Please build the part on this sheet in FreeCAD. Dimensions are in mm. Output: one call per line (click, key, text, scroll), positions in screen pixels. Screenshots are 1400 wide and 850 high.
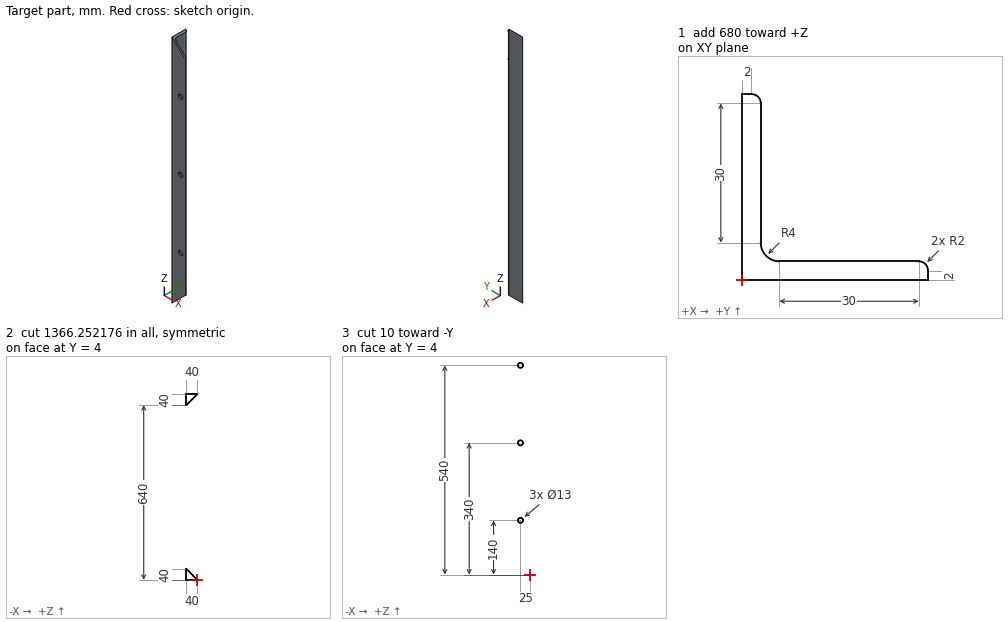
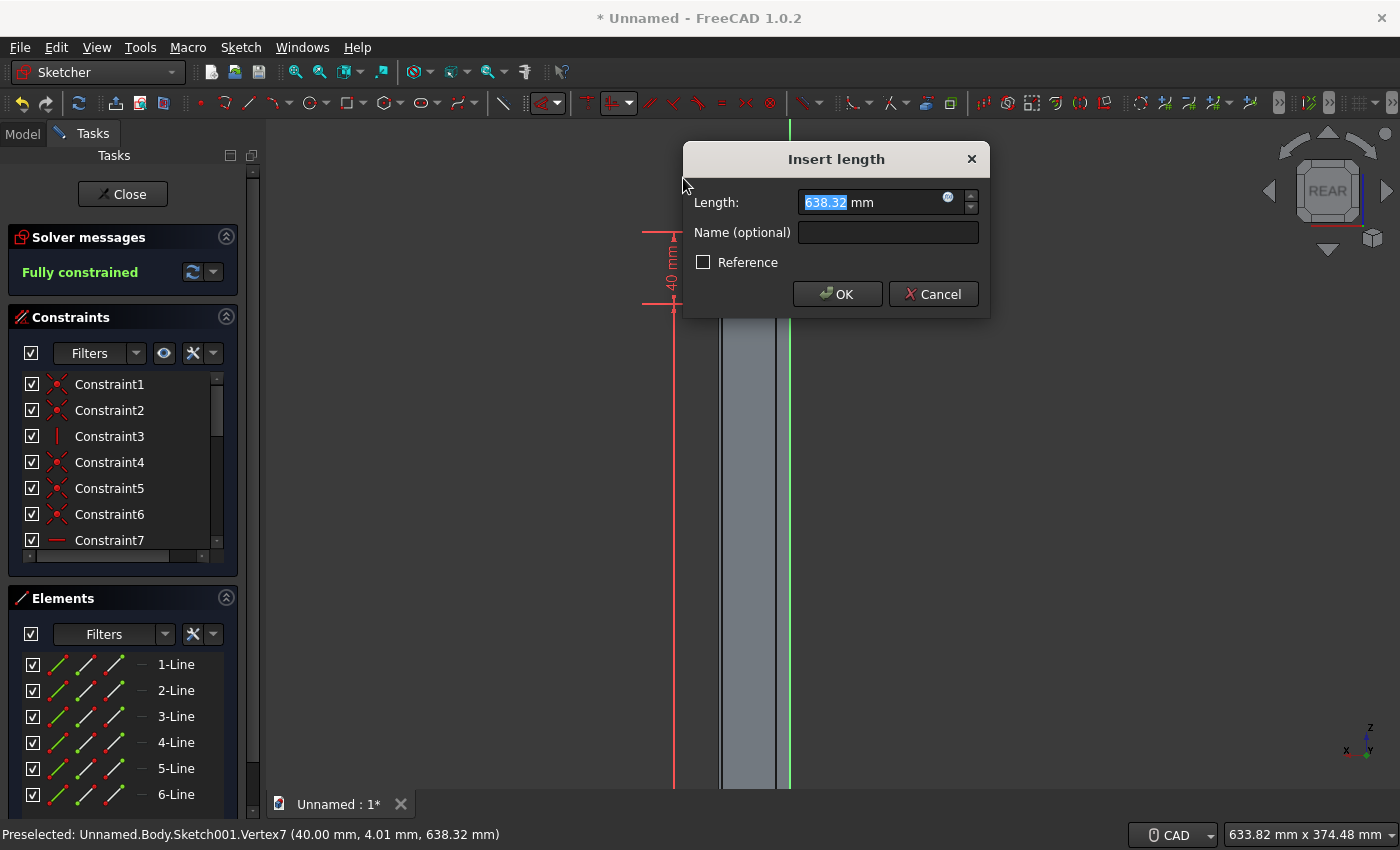
text(640)
key(Return)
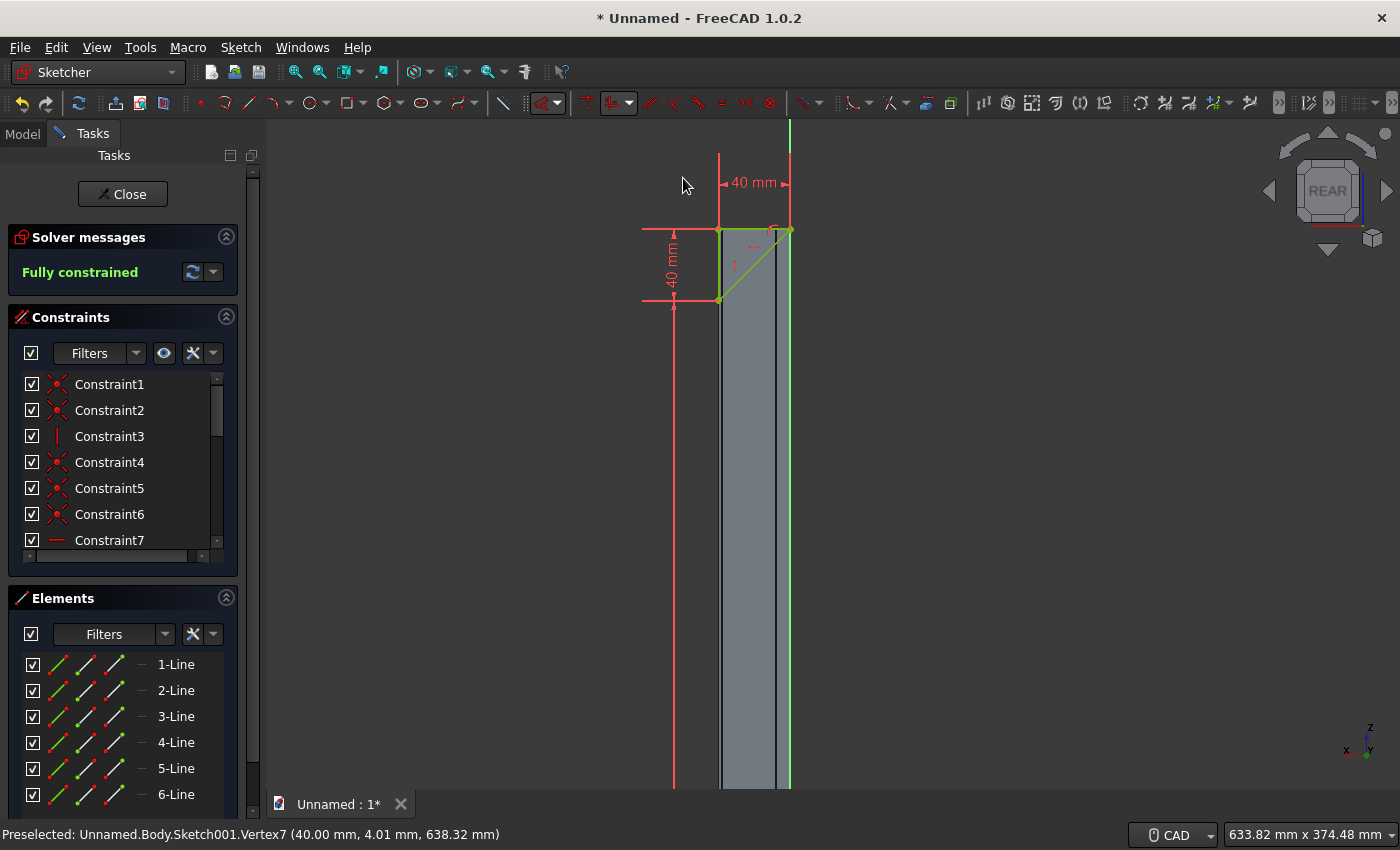
click(123, 194)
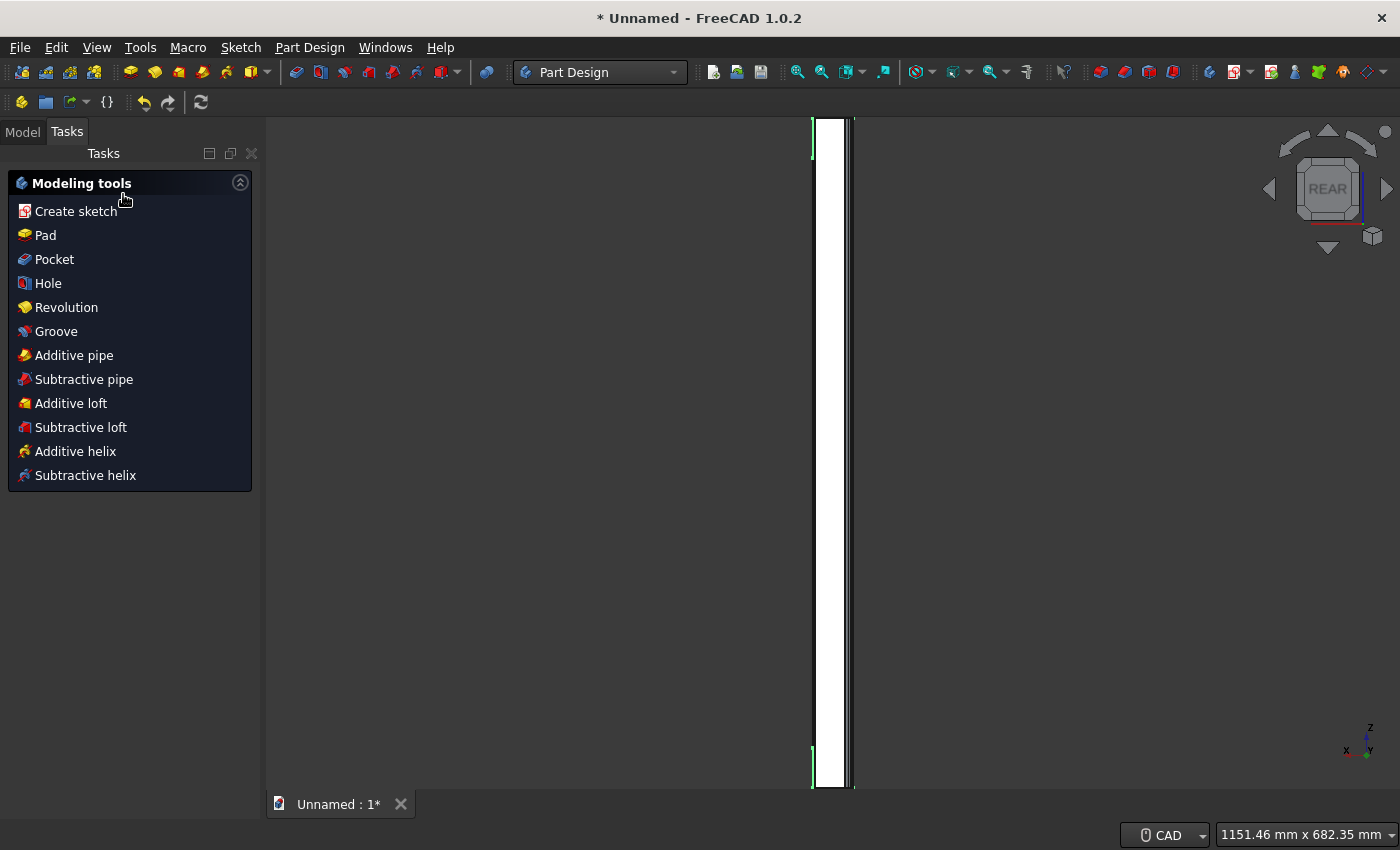
click(298, 72)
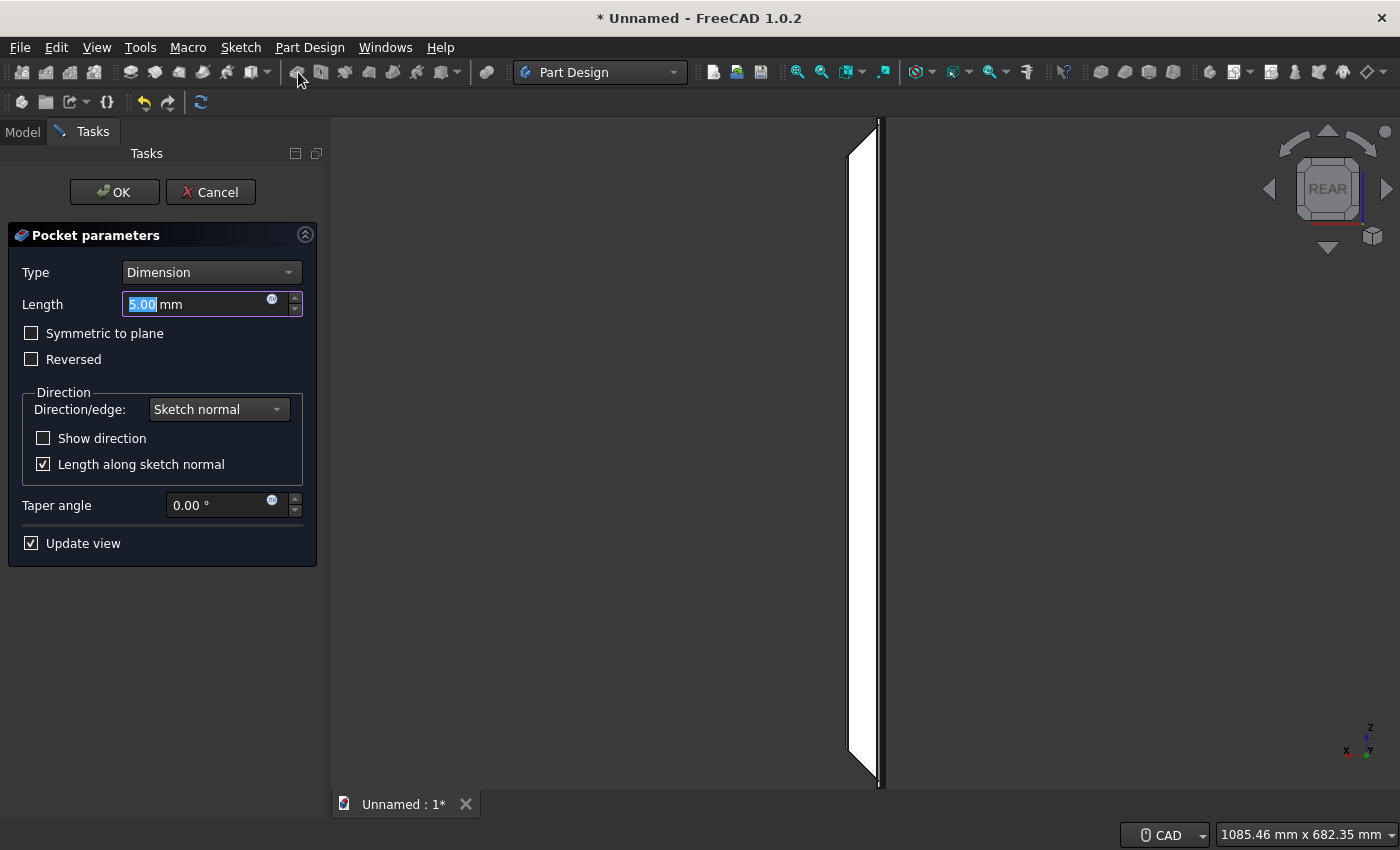
text(1366.252176)
key(Tab)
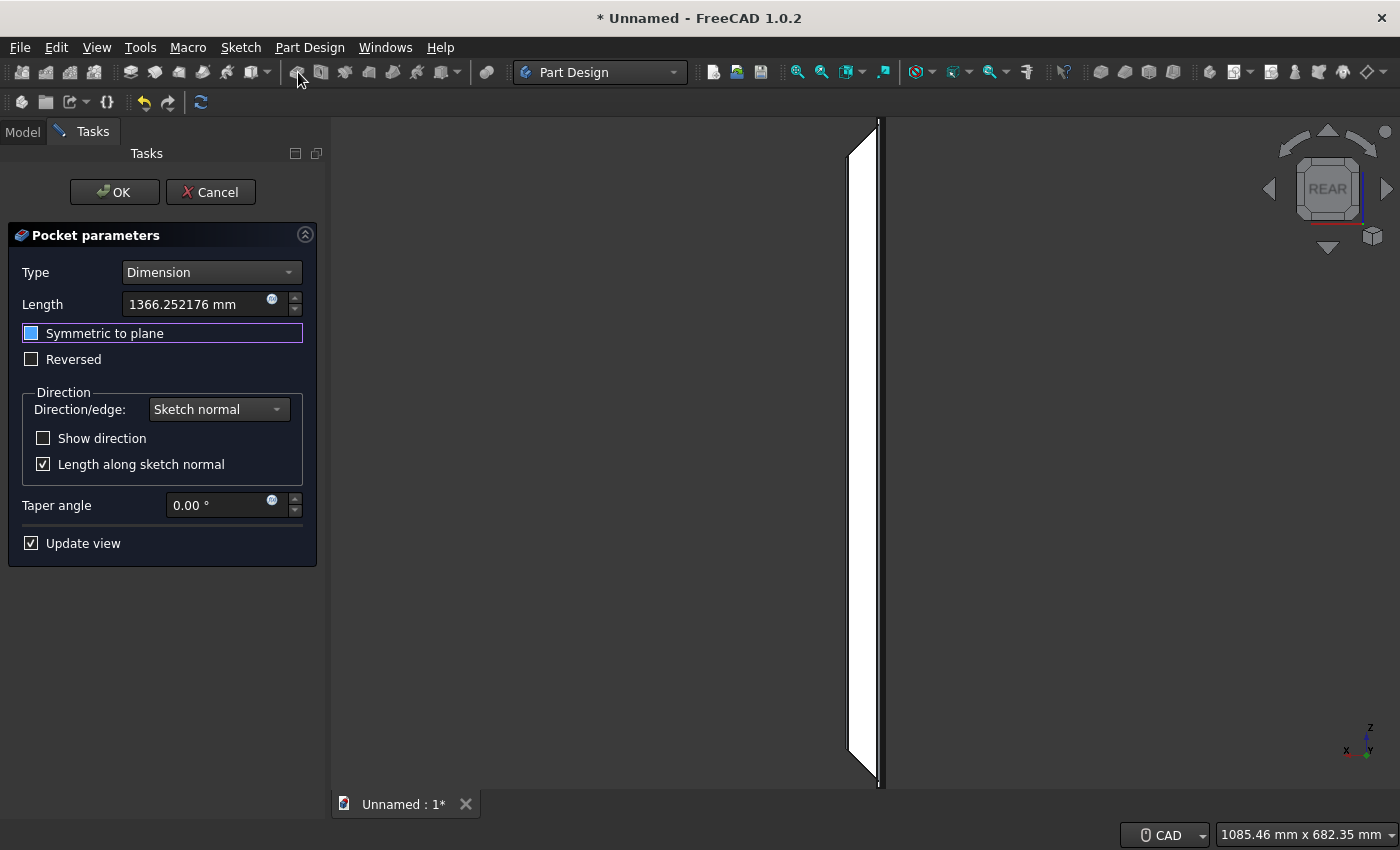
click(30, 333)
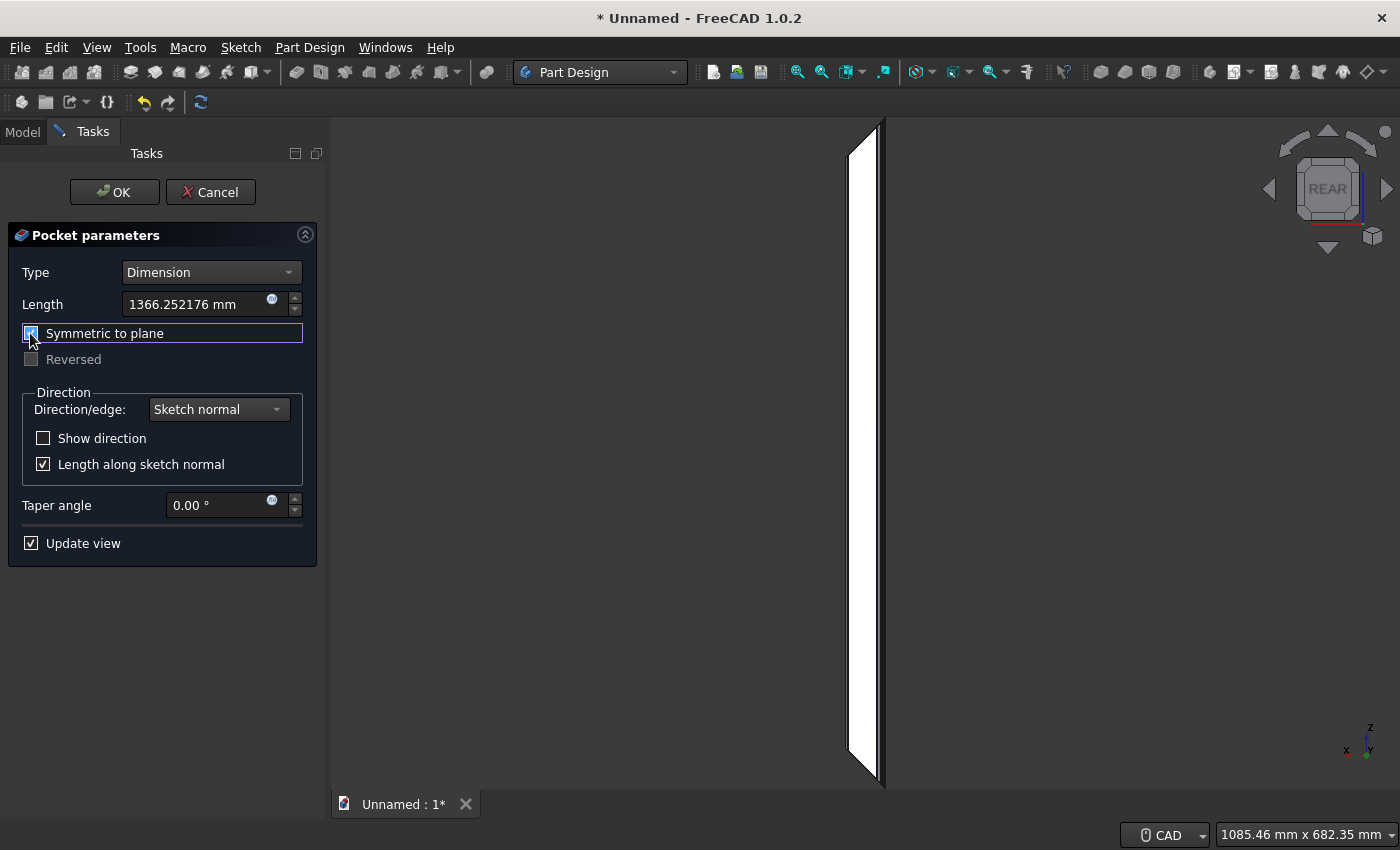
click(115, 192)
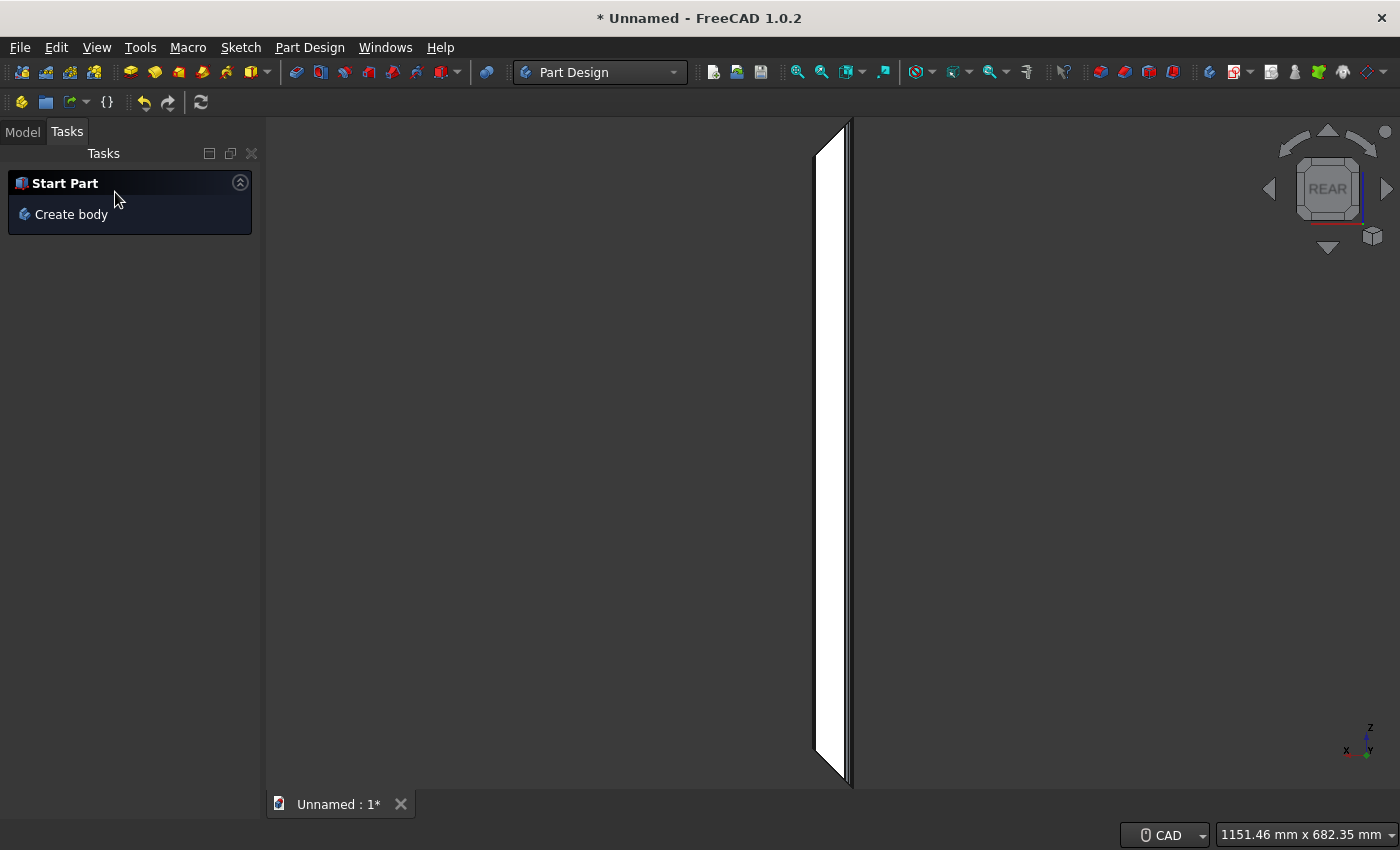
click(830, 172)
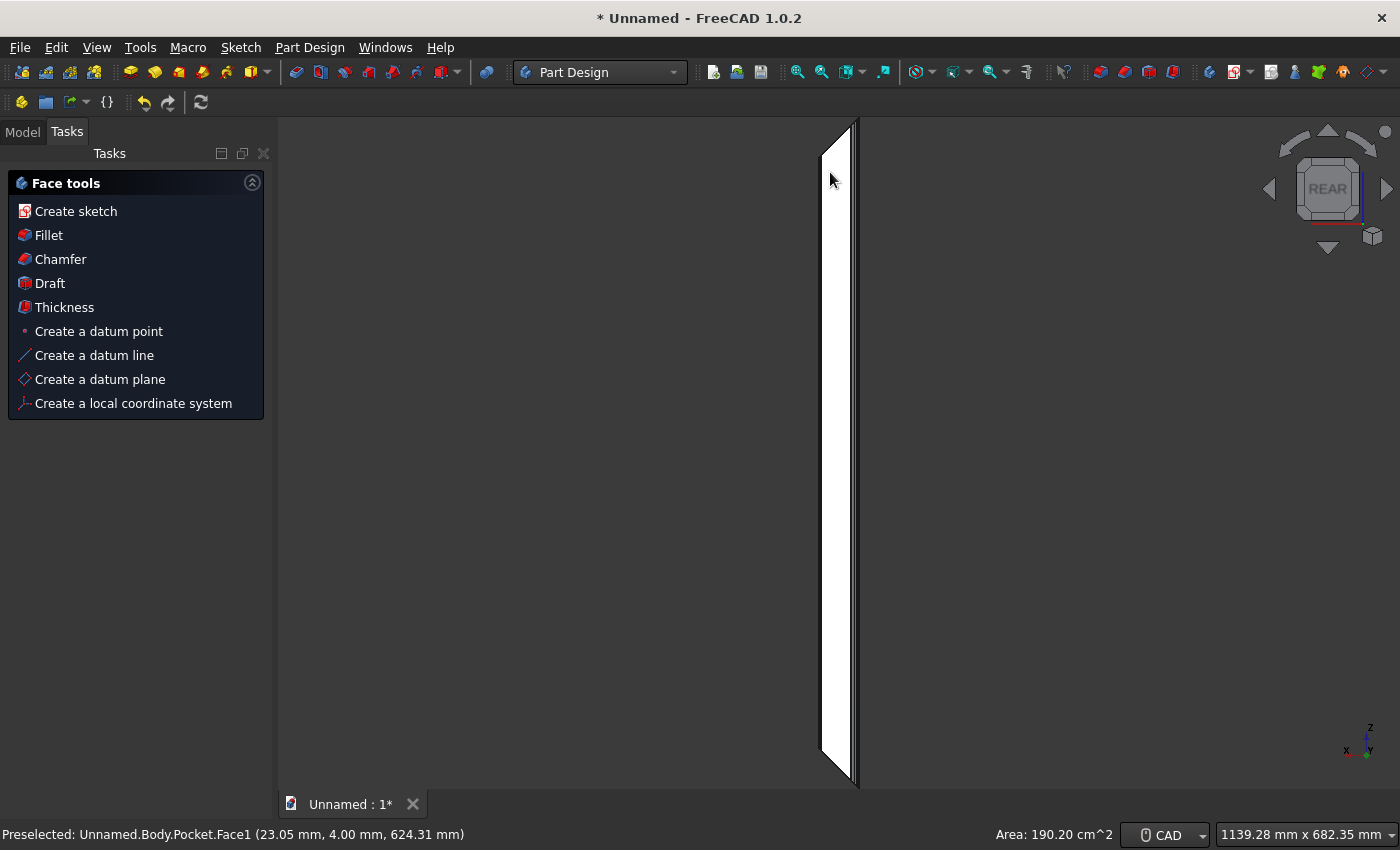
click(1234, 72)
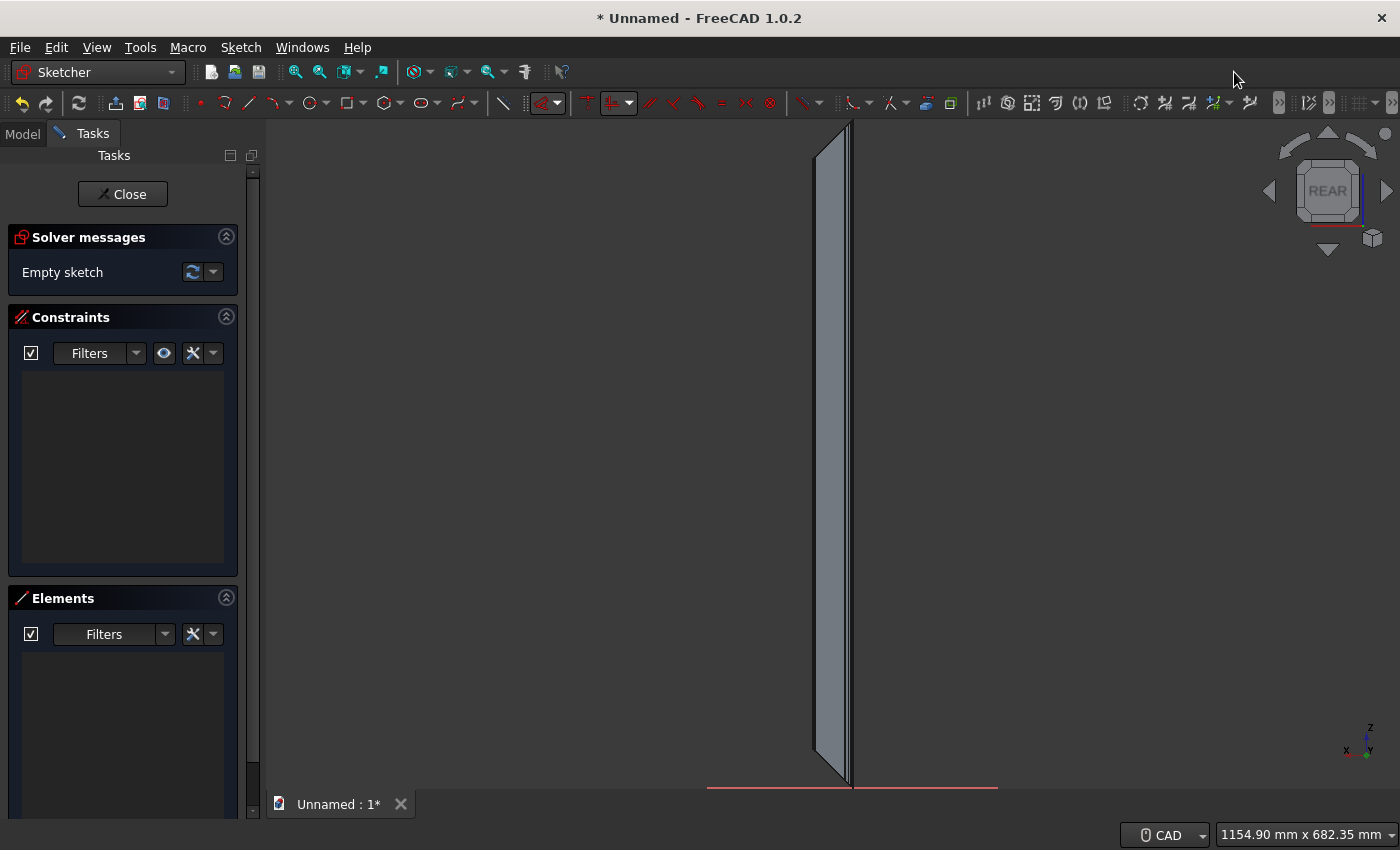
scroll(436, 158, down, 1)